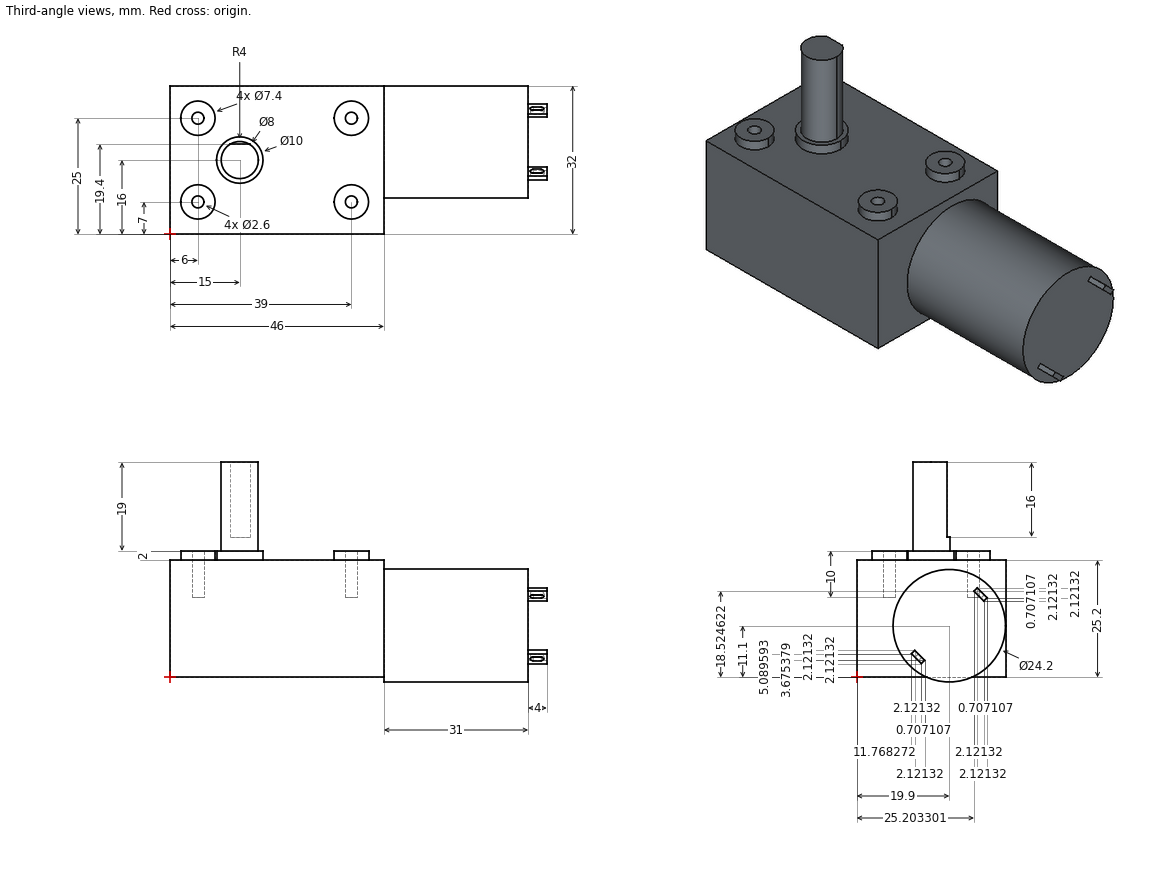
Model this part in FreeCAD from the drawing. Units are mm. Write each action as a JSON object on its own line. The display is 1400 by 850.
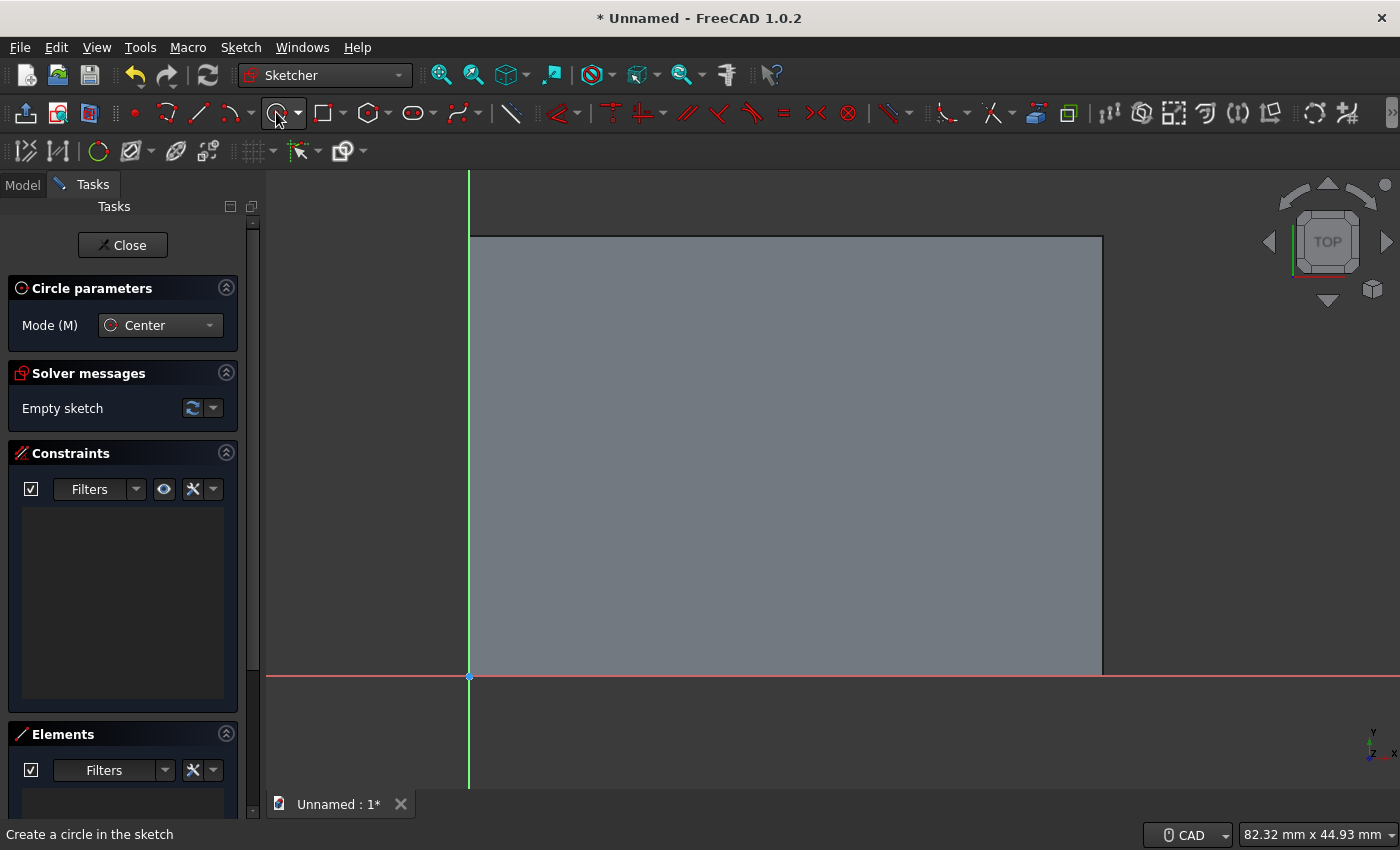
{"action": "left_click", "coordinate": [552, 332]}
{"action": "mouse_move", "coordinate": [588, 296]}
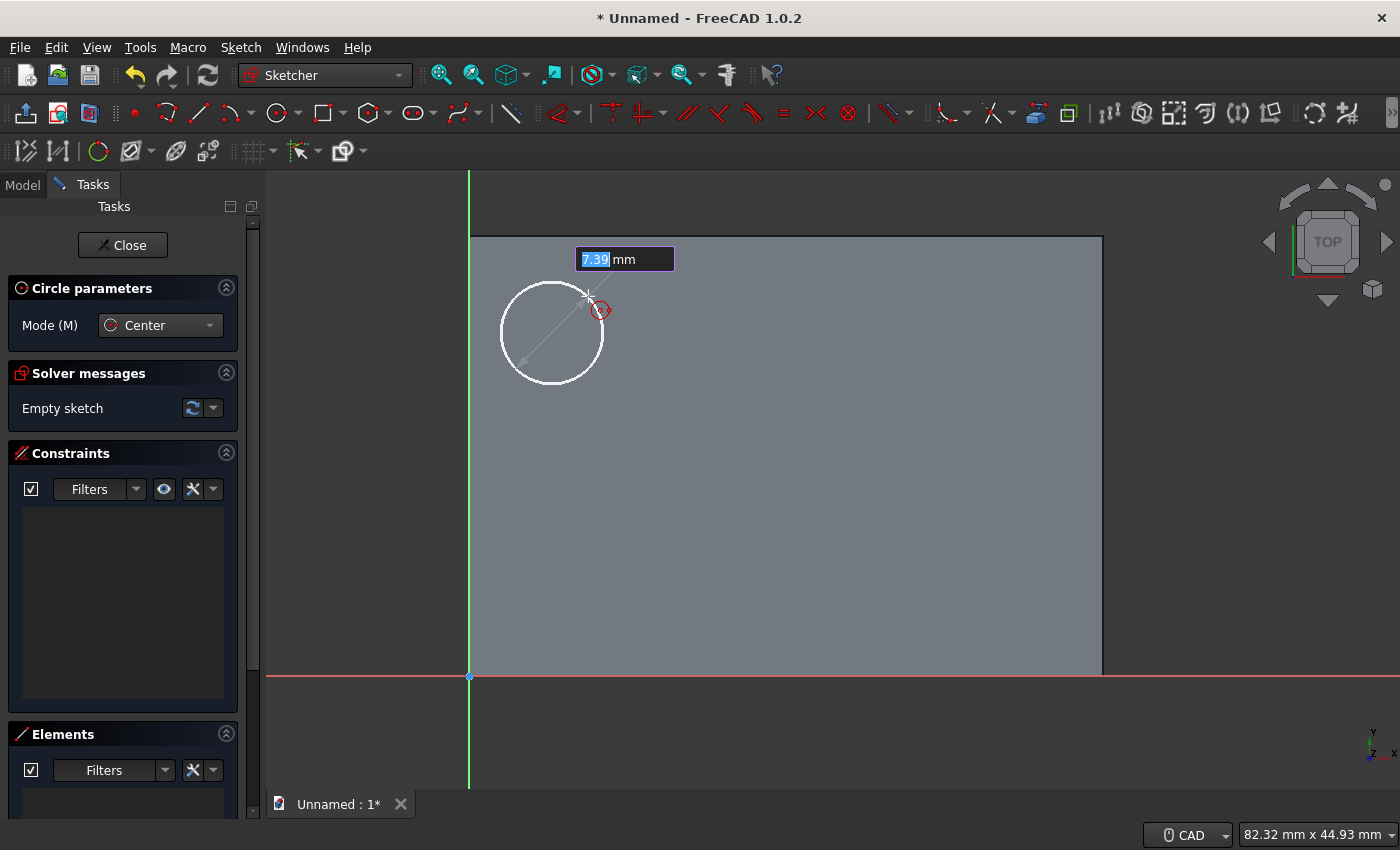
{"action": "type", "text": "7.4"}
{"action": "key", "text": "Return"}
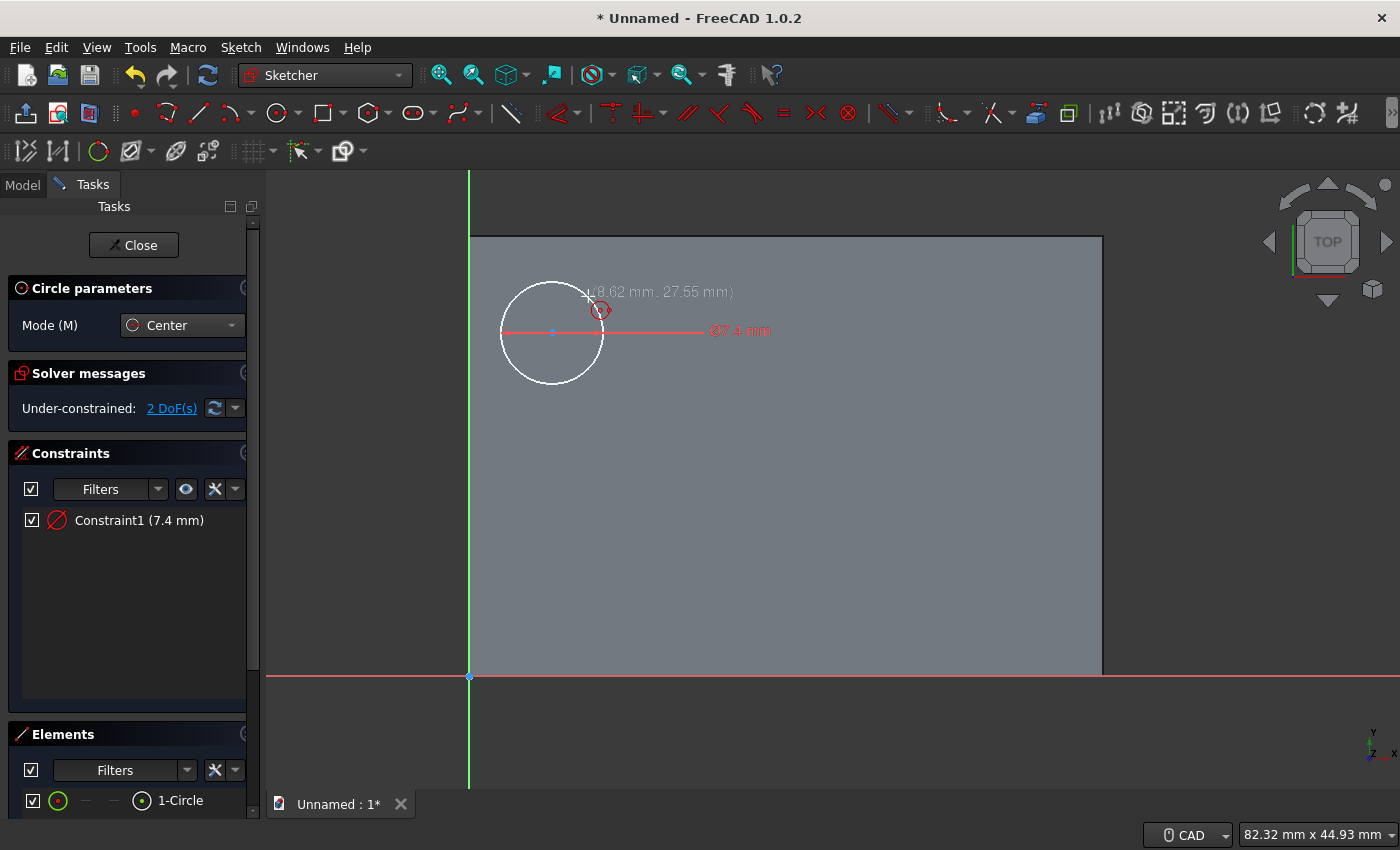
{"action": "left_click", "coordinate": [552, 580]}
{"action": "mouse_move", "coordinate": [588, 544]}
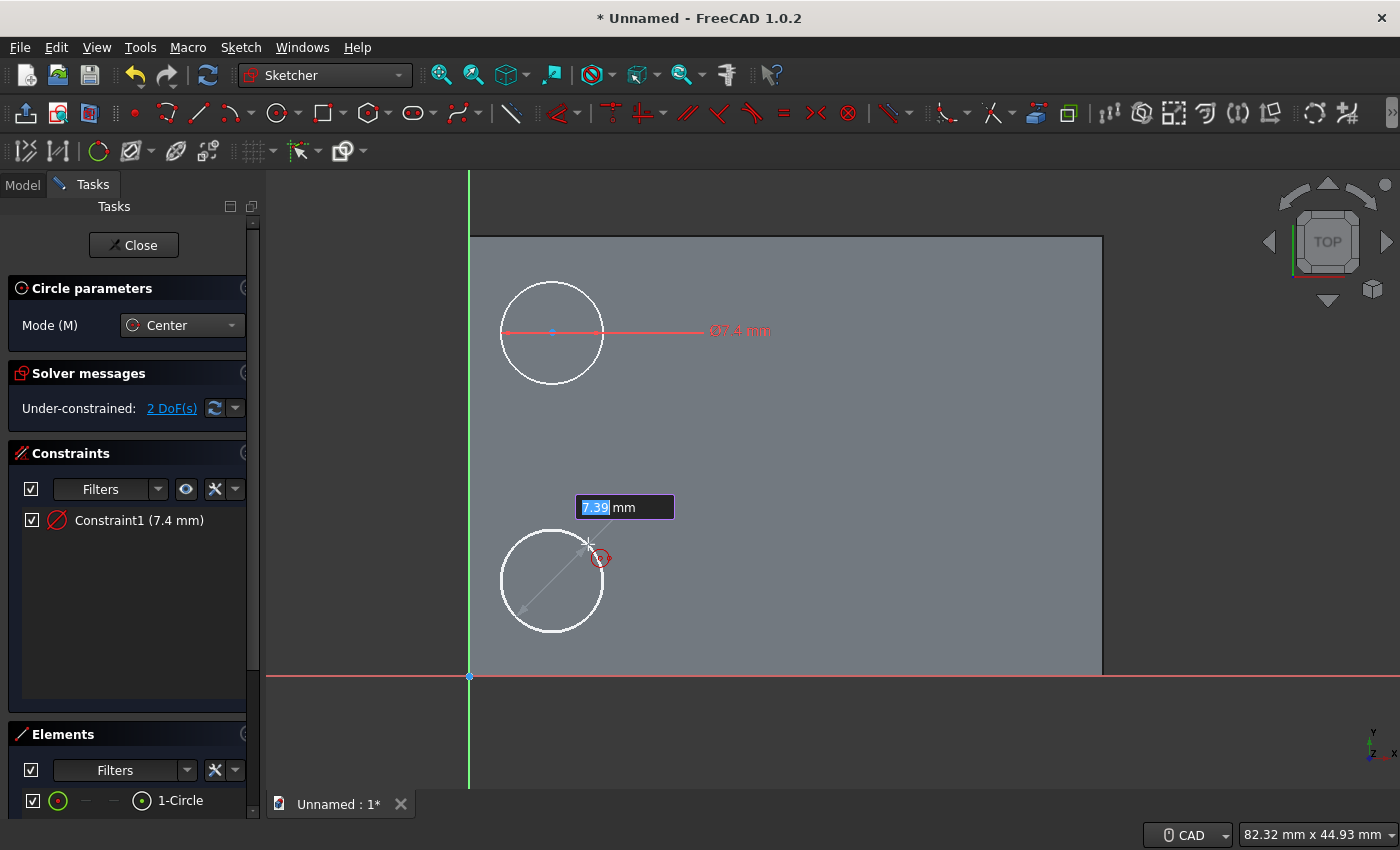
{"action": "type", "text": "7.4"}
{"action": "key", "text": "Return"}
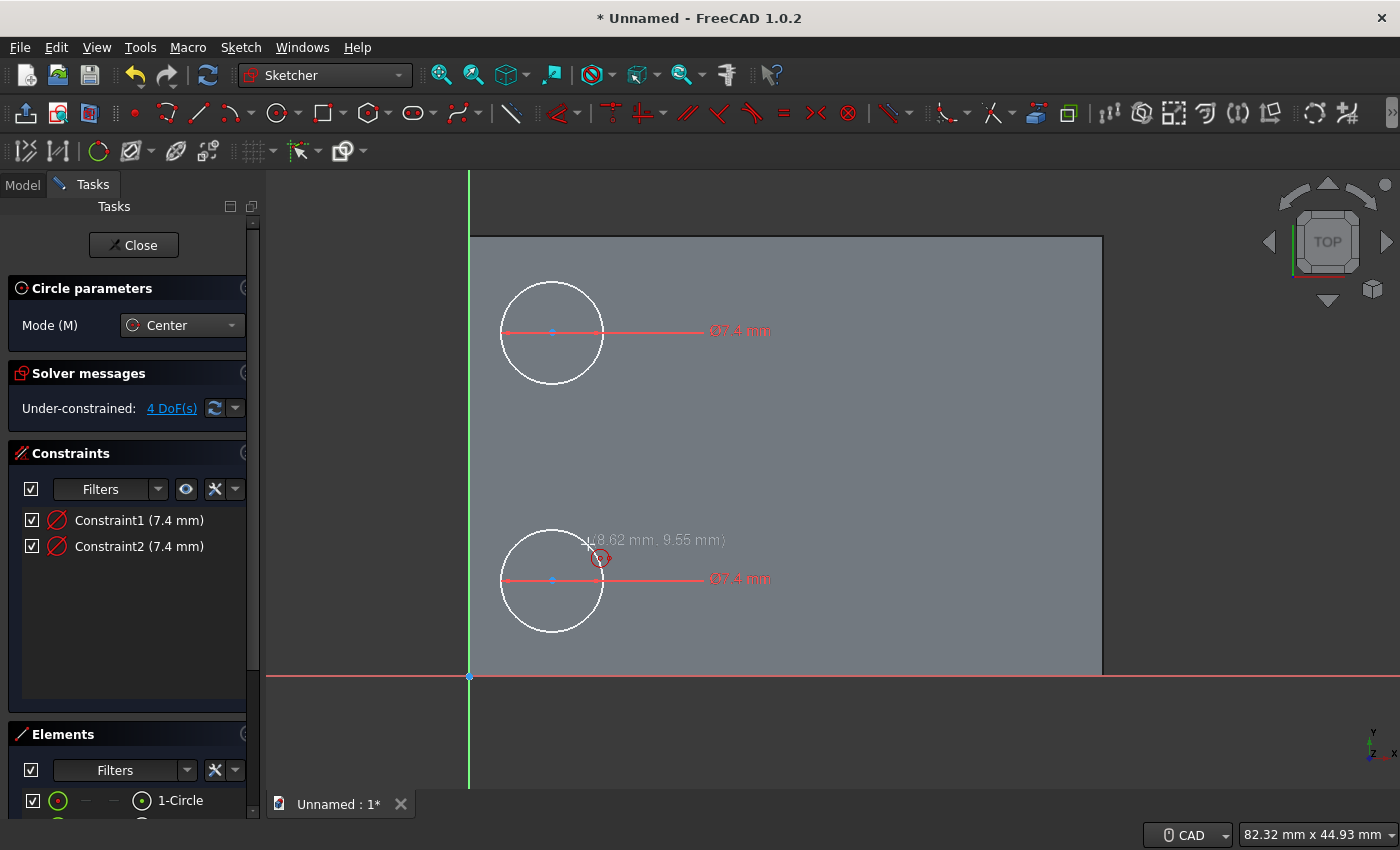
{"action": "left_click", "coordinate": [1007, 580]}
{"action": "mouse_move", "coordinate": [1043, 544]}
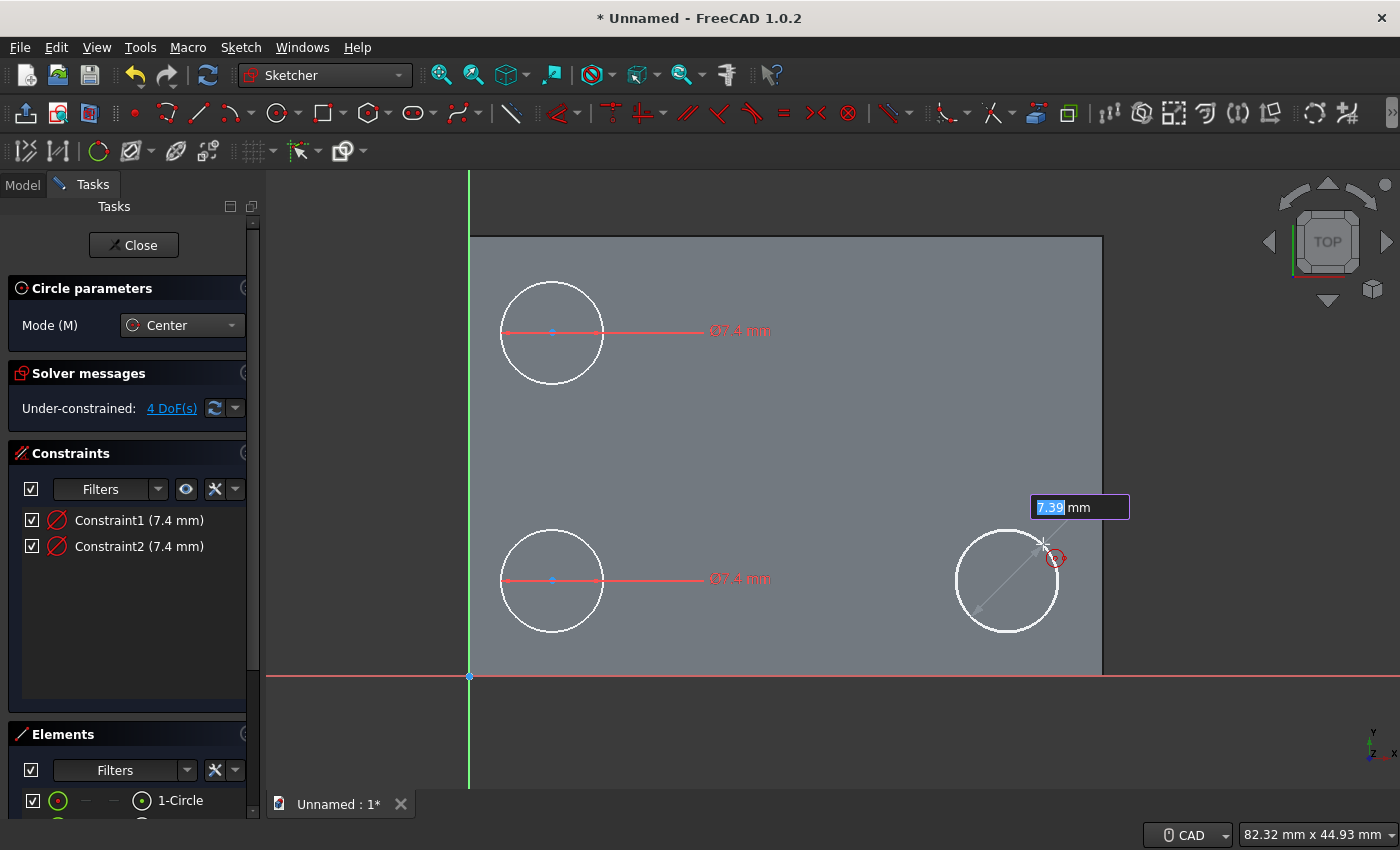
{"action": "type", "text": "7.4"}
{"action": "key", "text": "Return"}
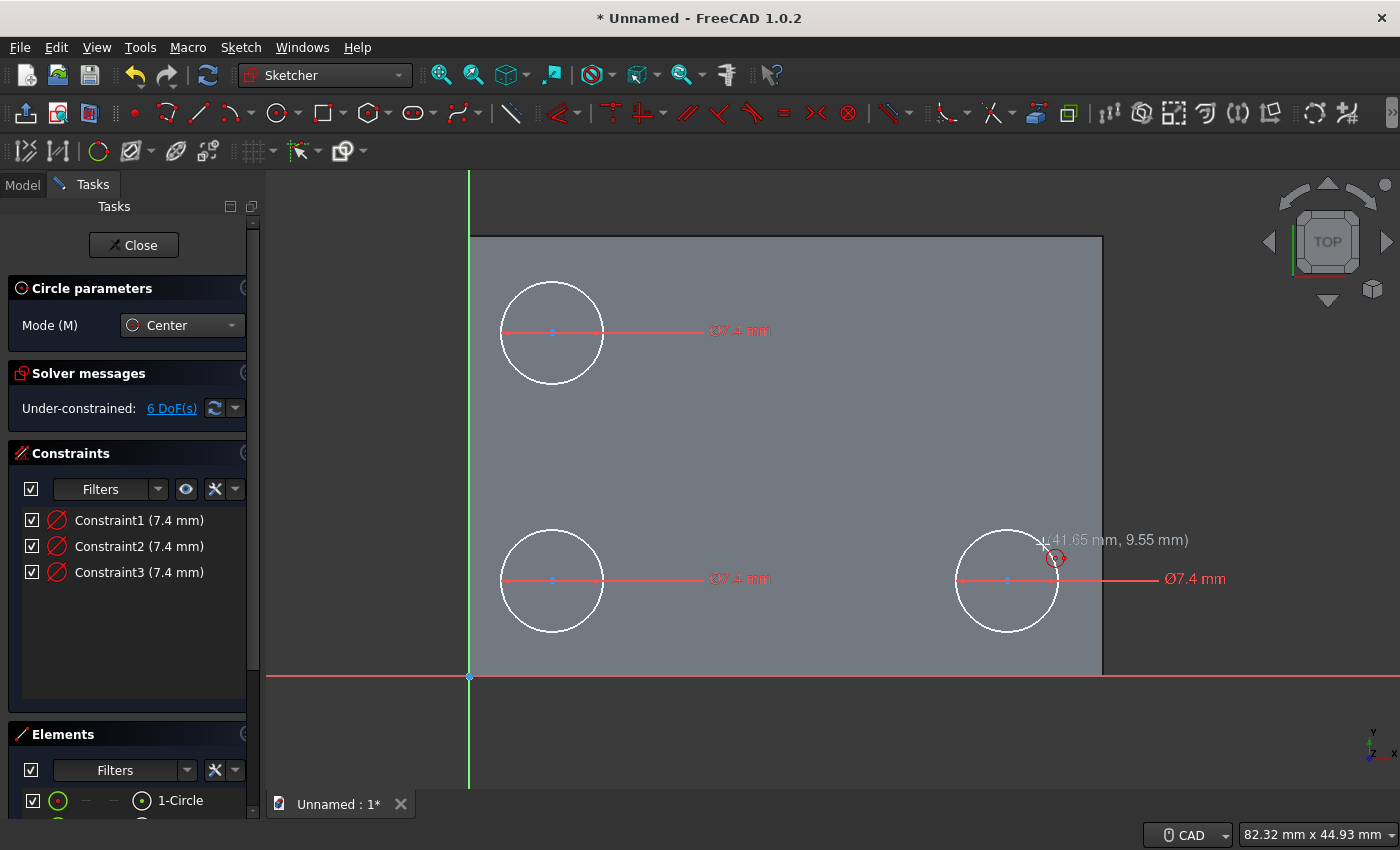
{"action": "left_click", "coordinate": [1007, 332]}
{"action": "mouse_move", "coordinate": [1043, 296]}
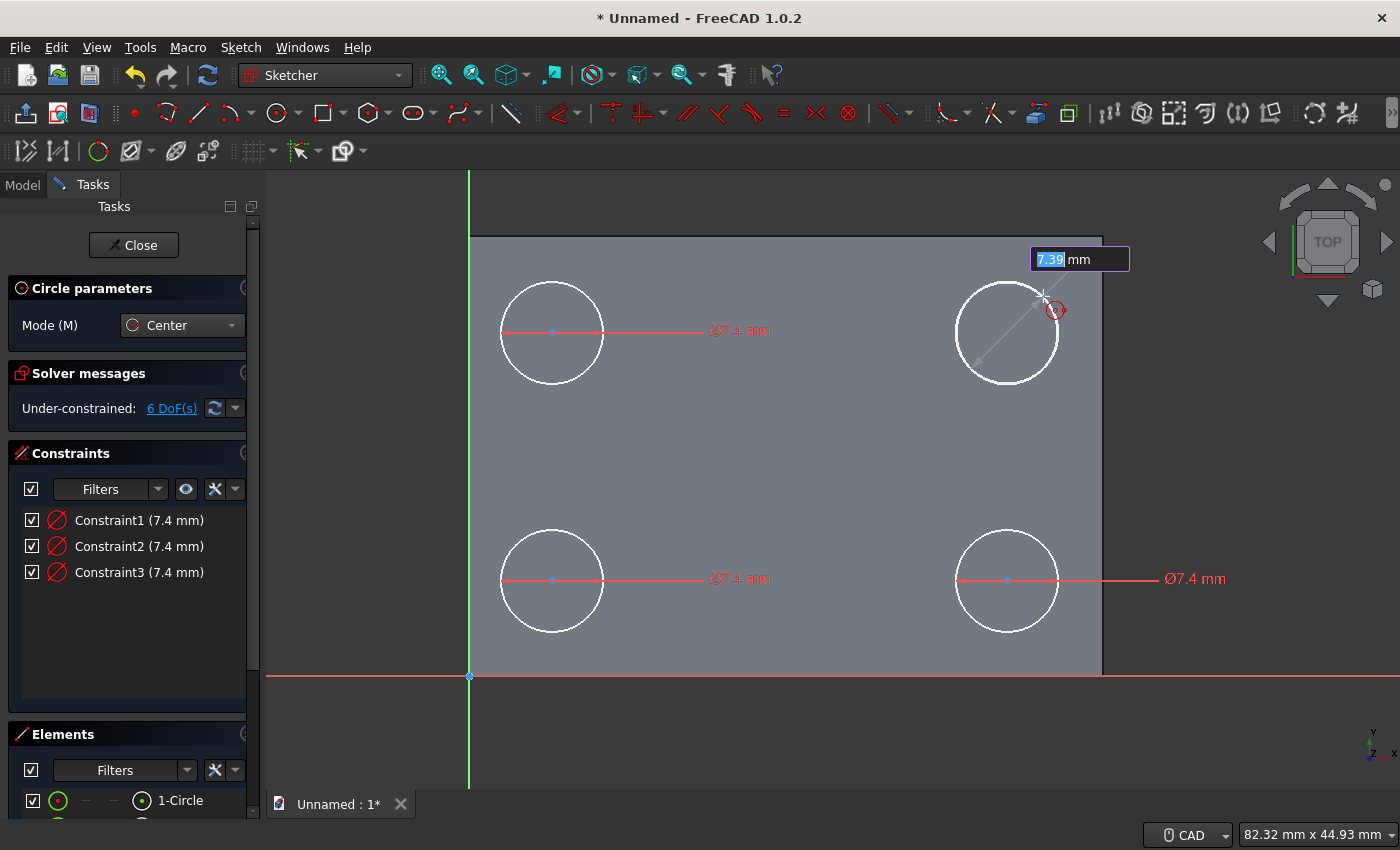
{"action": "type", "text": "7.4"}
{"action": "key", "text": "Return"}